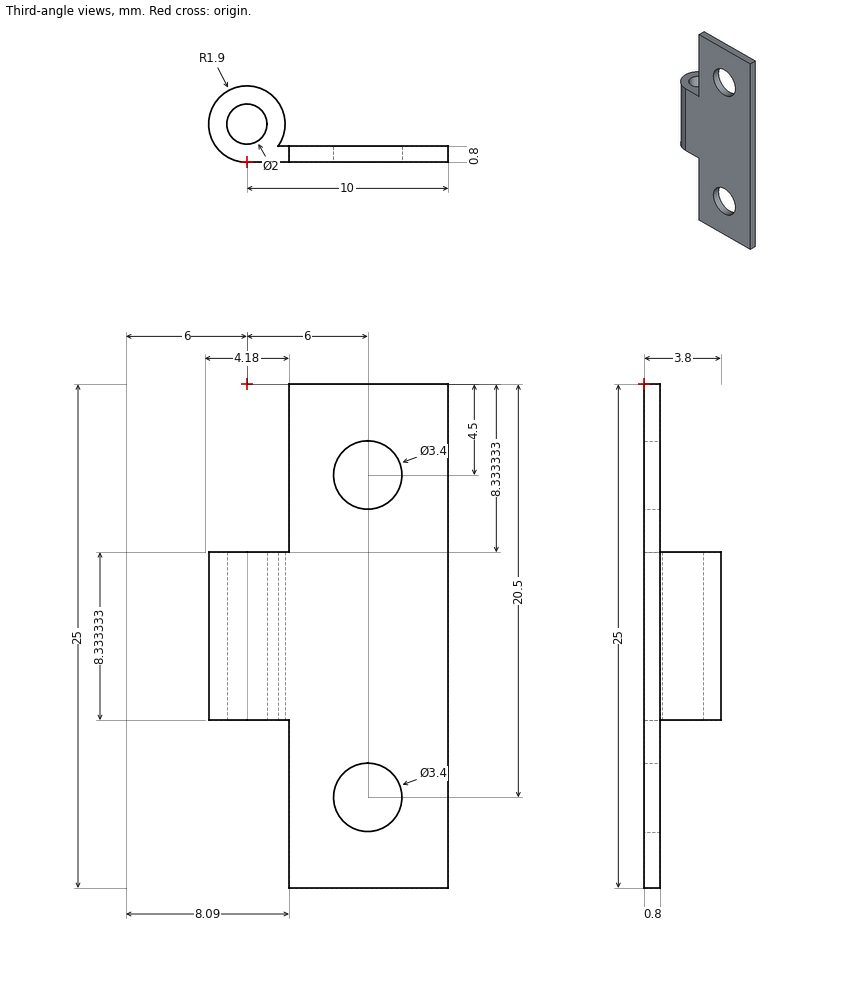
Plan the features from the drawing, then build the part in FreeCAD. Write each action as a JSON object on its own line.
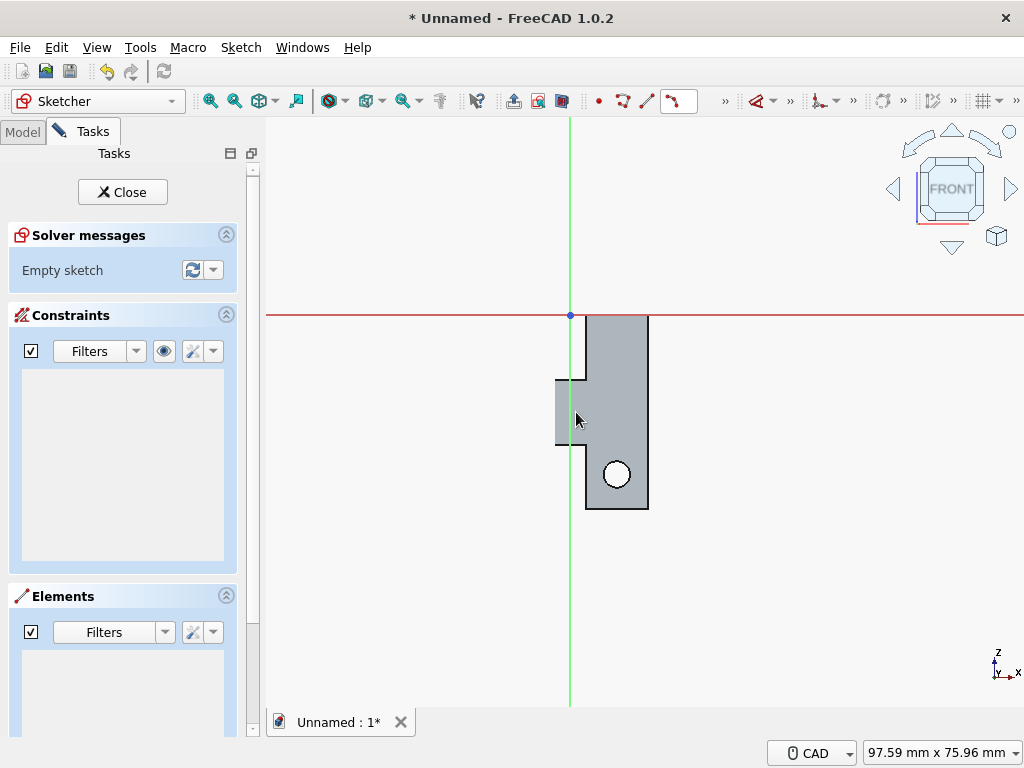
{"action": "scroll", "coordinate": [605, 325], "scroll_direction": "up", "scroll_amount": 9}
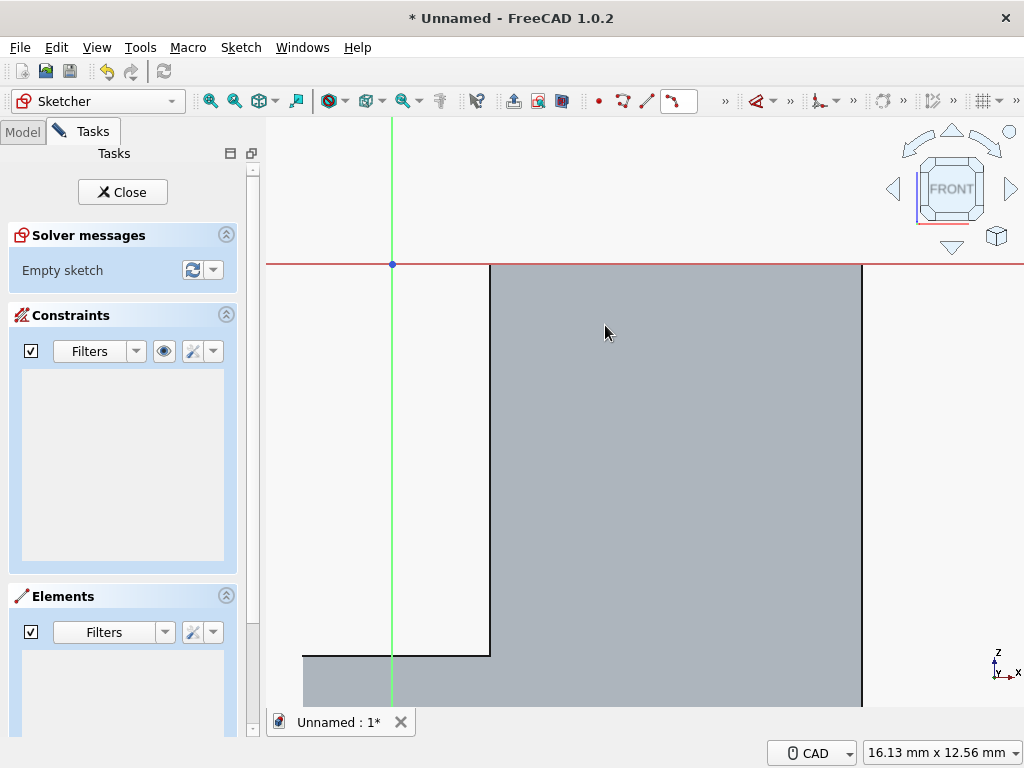
{"action": "key", "text": "g c"}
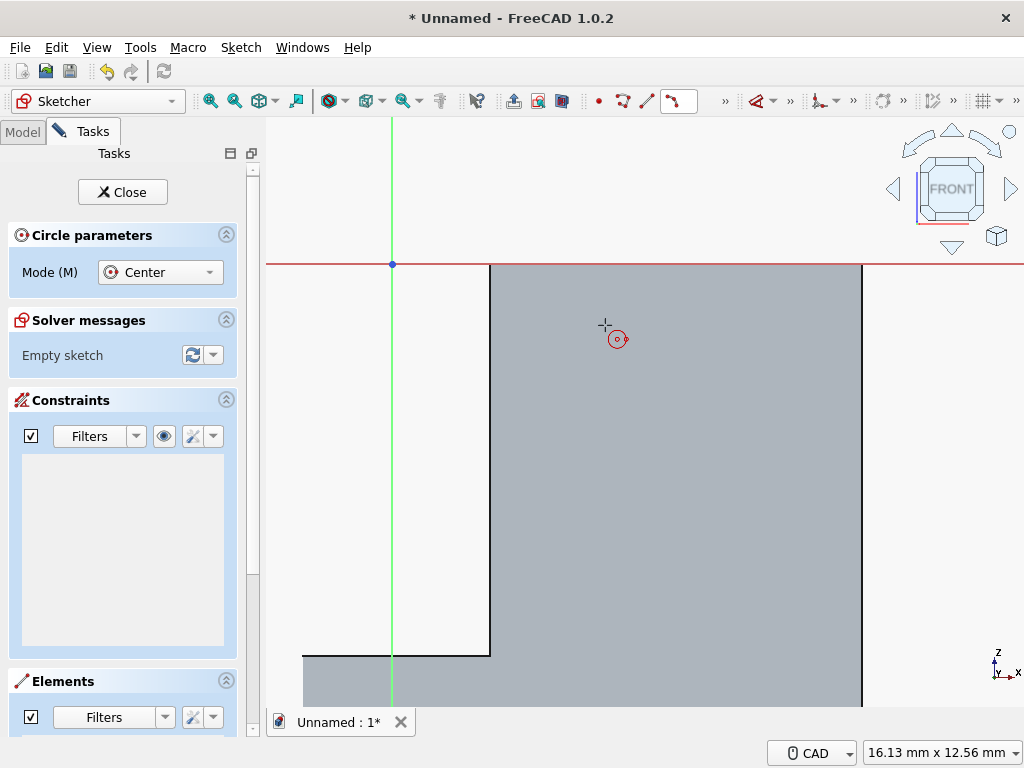
{"action": "left_click", "coordinate": [674, 476]}
{"action": "left_click", "coordinate": [730, 419]}
{"action": "key", "text": "Escape"}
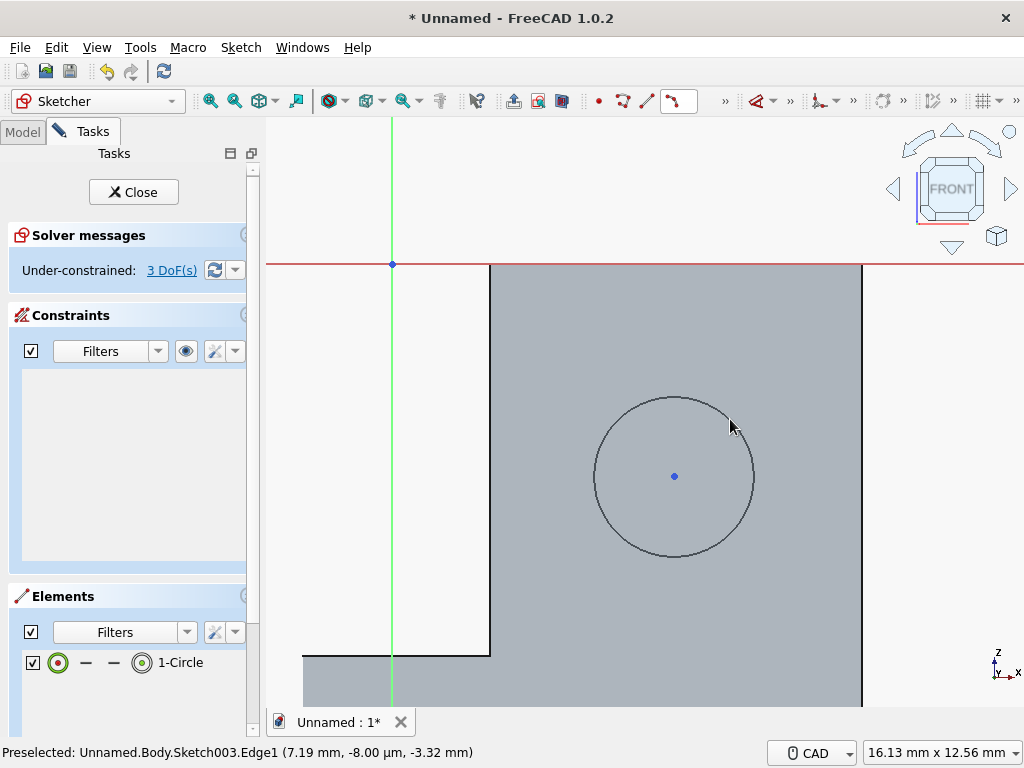
{"action": "left_click", "coordinate": [756, 102]}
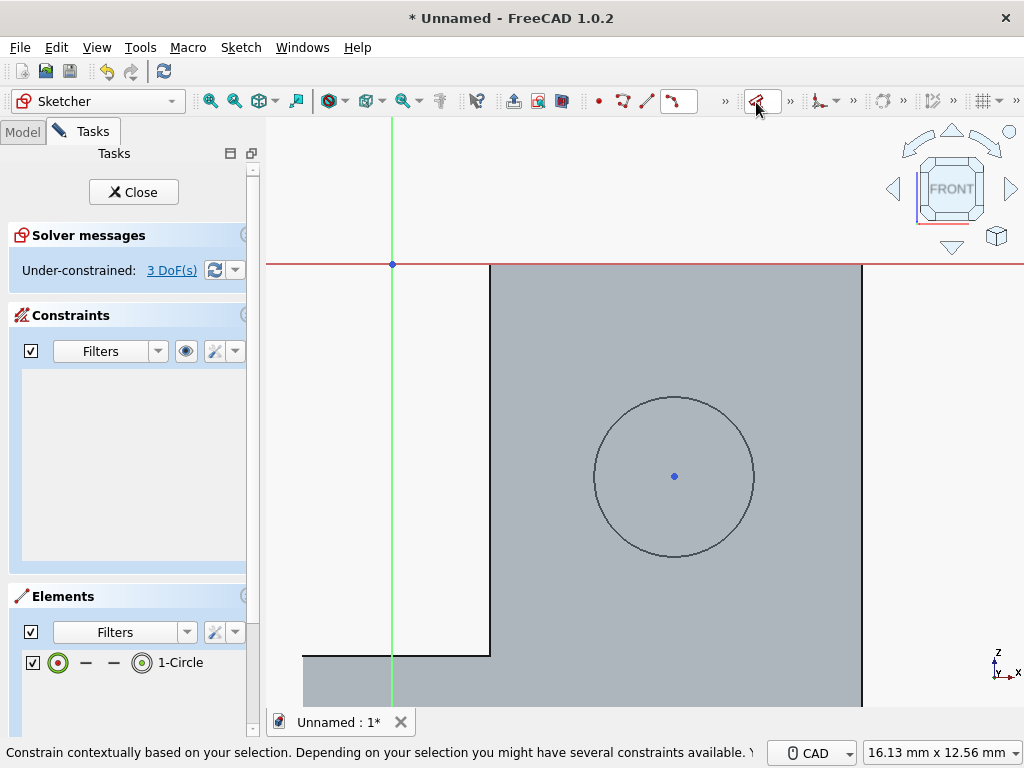
{"action": "left_click", "coordinate": [730, 420]}
{"action": "left_click", "coordinate": [752, 397]}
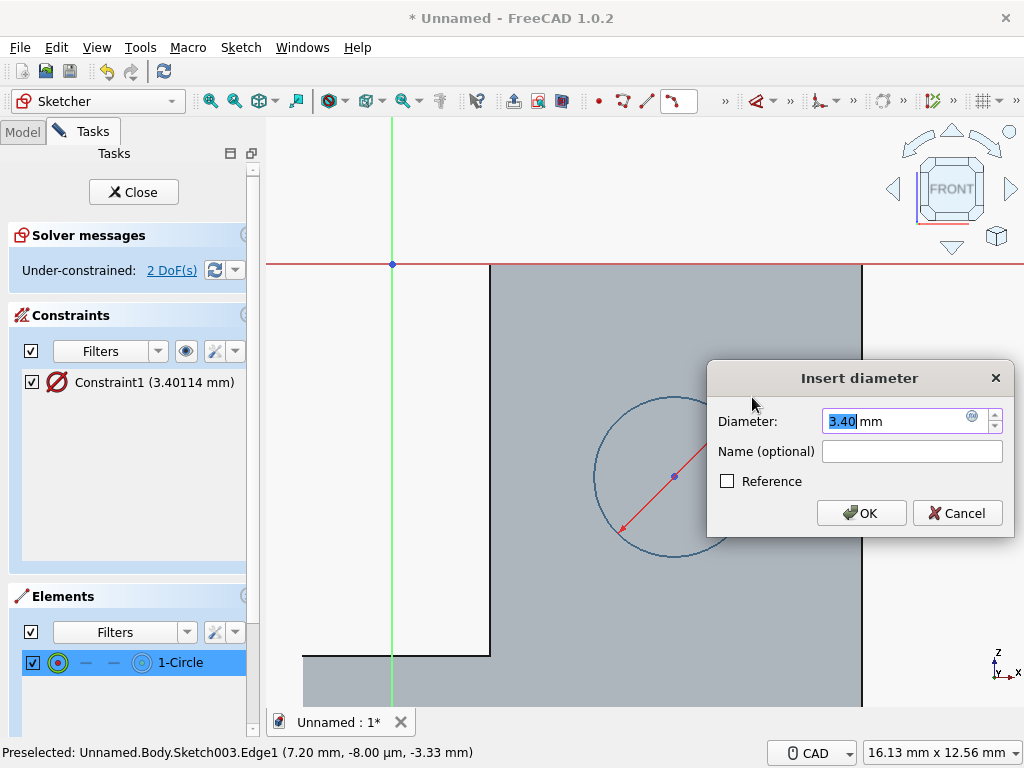
{"action": "type", "text": "3.4"}
{"action": "key", "text": "Return"}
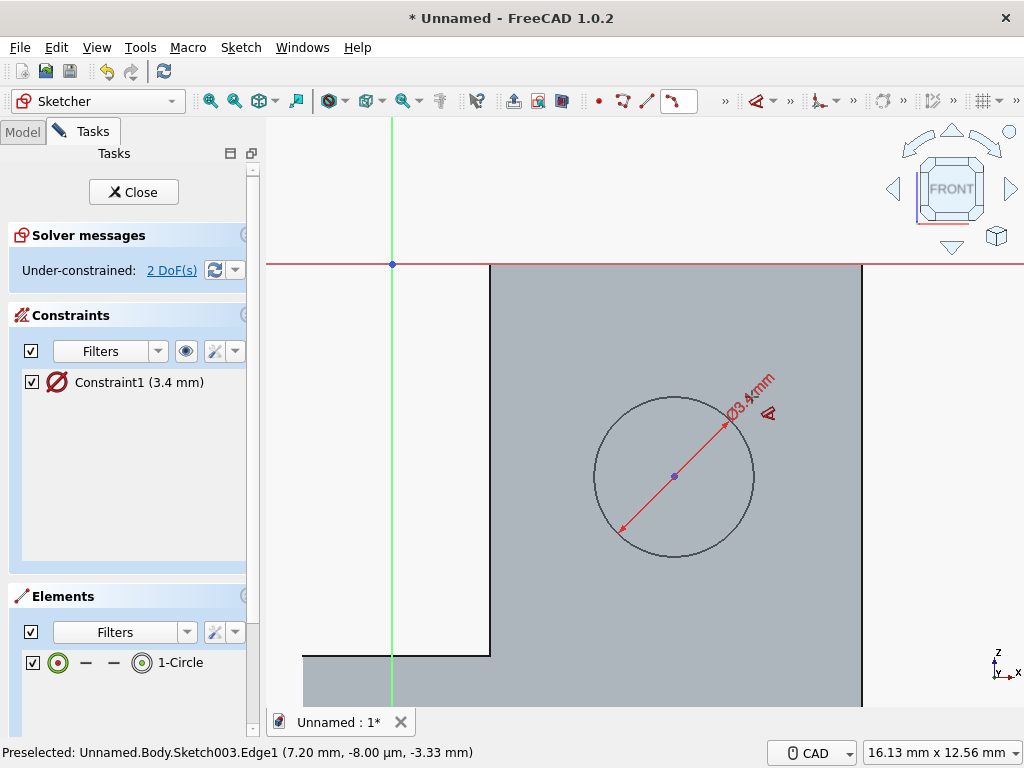
{"action": "left_click", "coordinate": [674, 477]}
{"action": "left_click", "coordinate": [533, 230]}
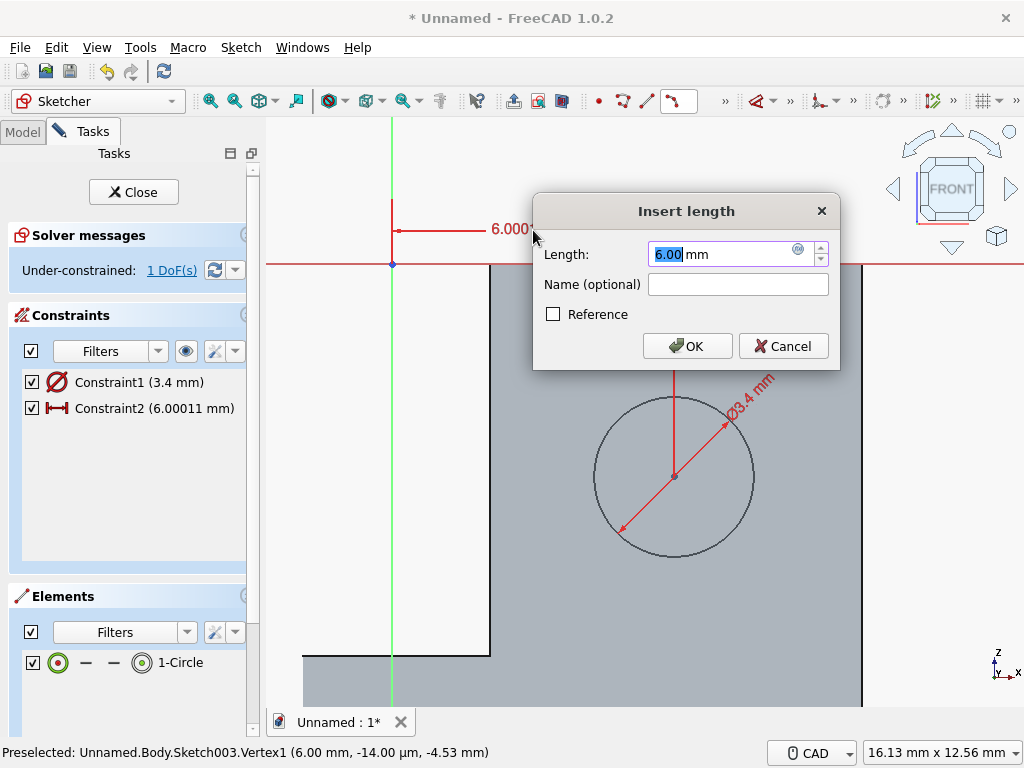
{"action": "type", "text": "6"}
{"action": "key", "text": "Return"}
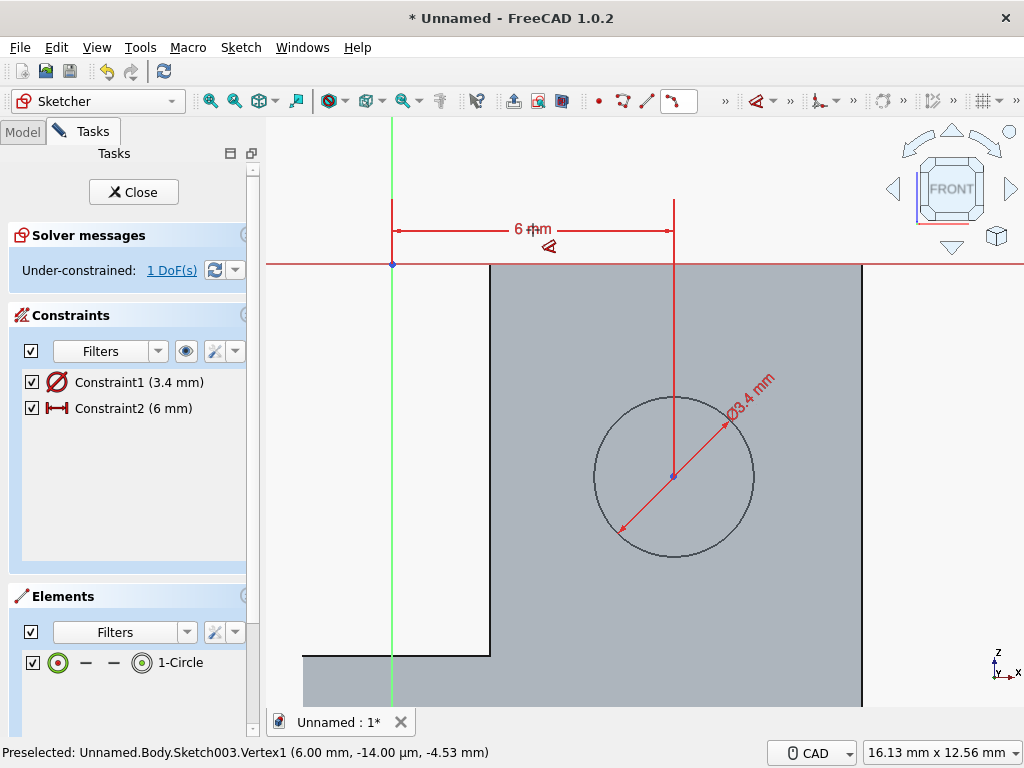
{"action": "left_click", "coordinate": [674, 477]}
{"action": "left_click", "coordinate": [358, 371]}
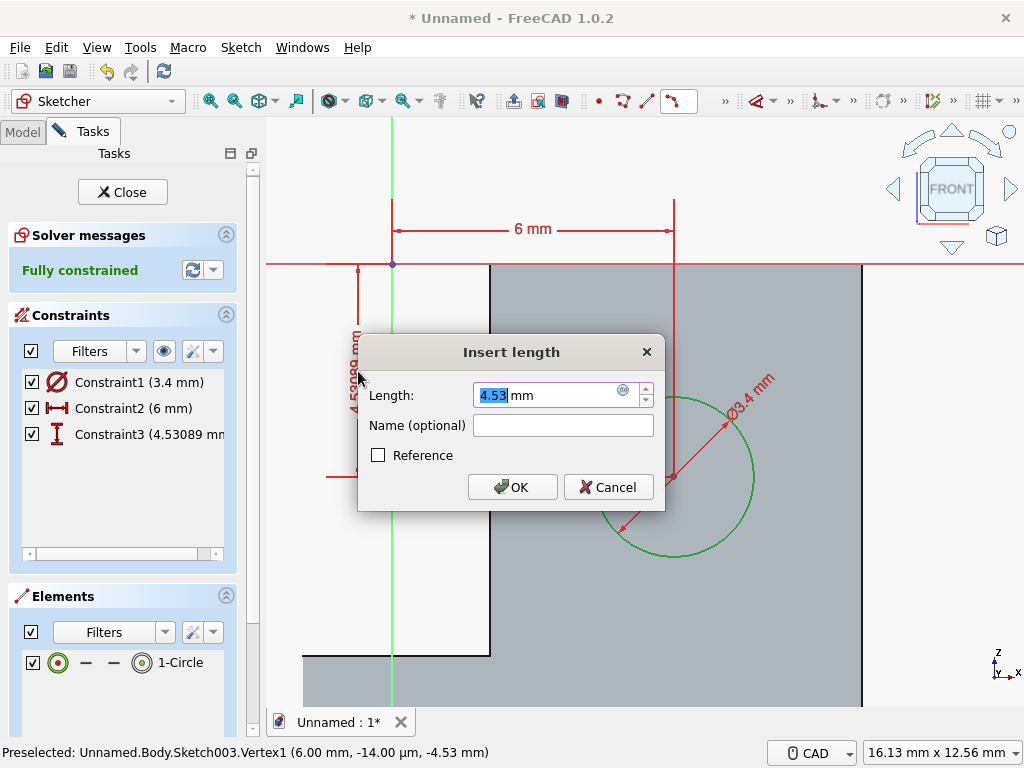
{"action": "type", "text": "4.5"}
{"action": "key", "text": "Return"}
{"action": "key", "text": "Escape"}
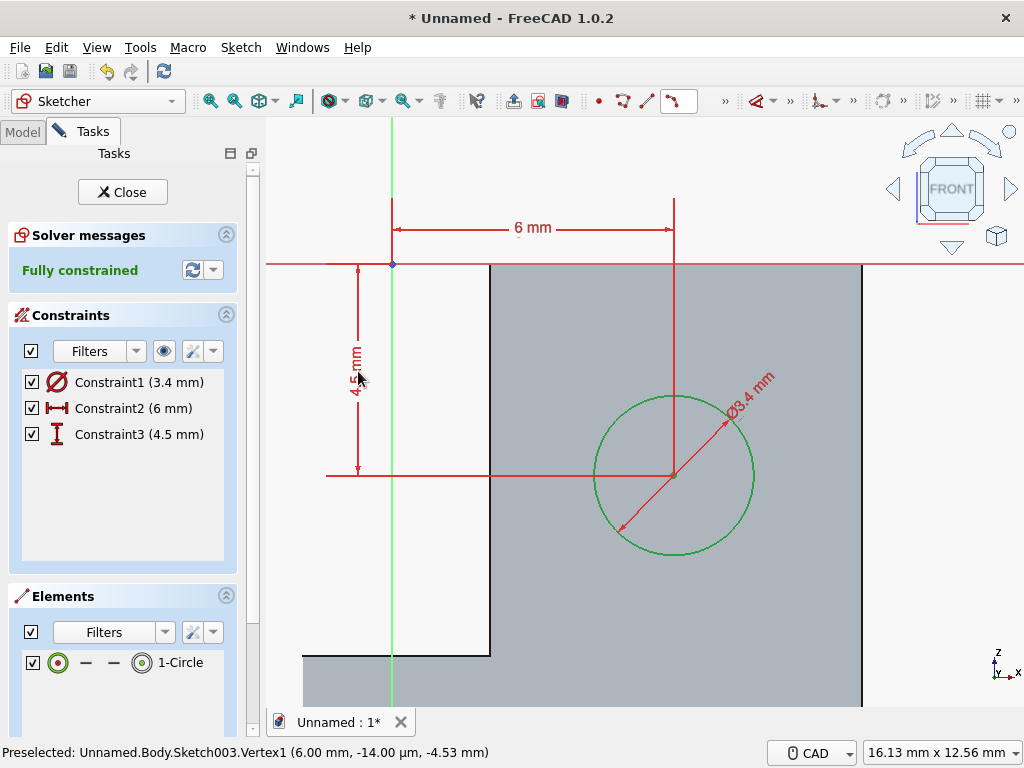
{"action": "left_click", "coordinate": [123, 192]}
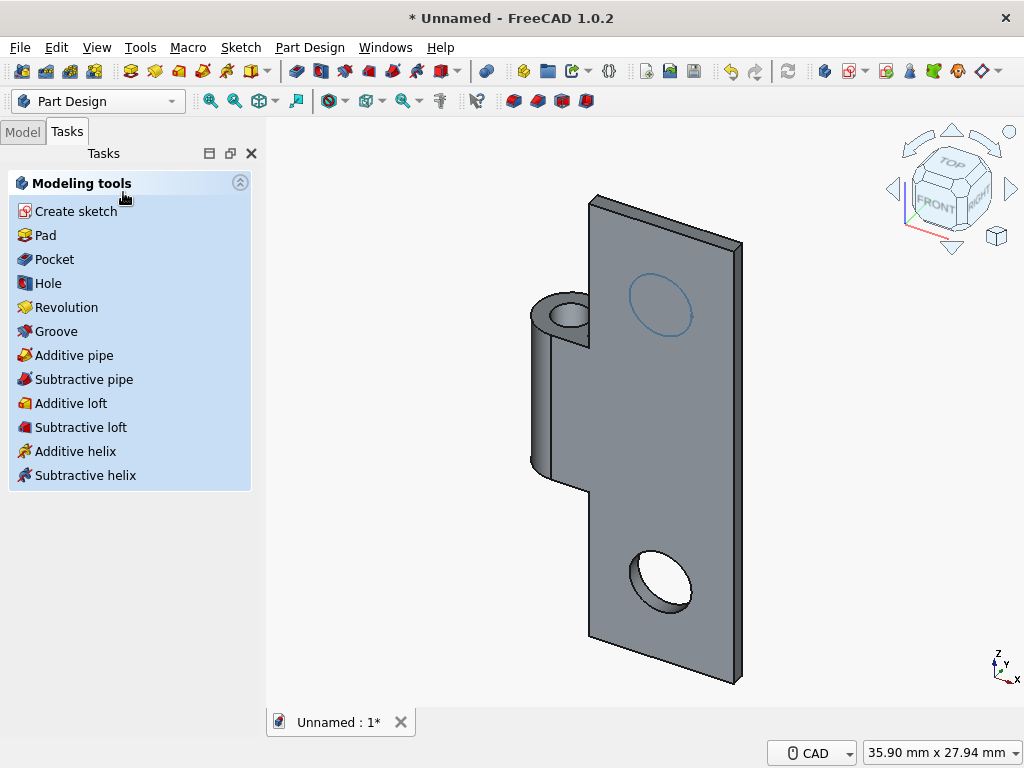
{"action": "left_click", "coordinate": [298, 72]}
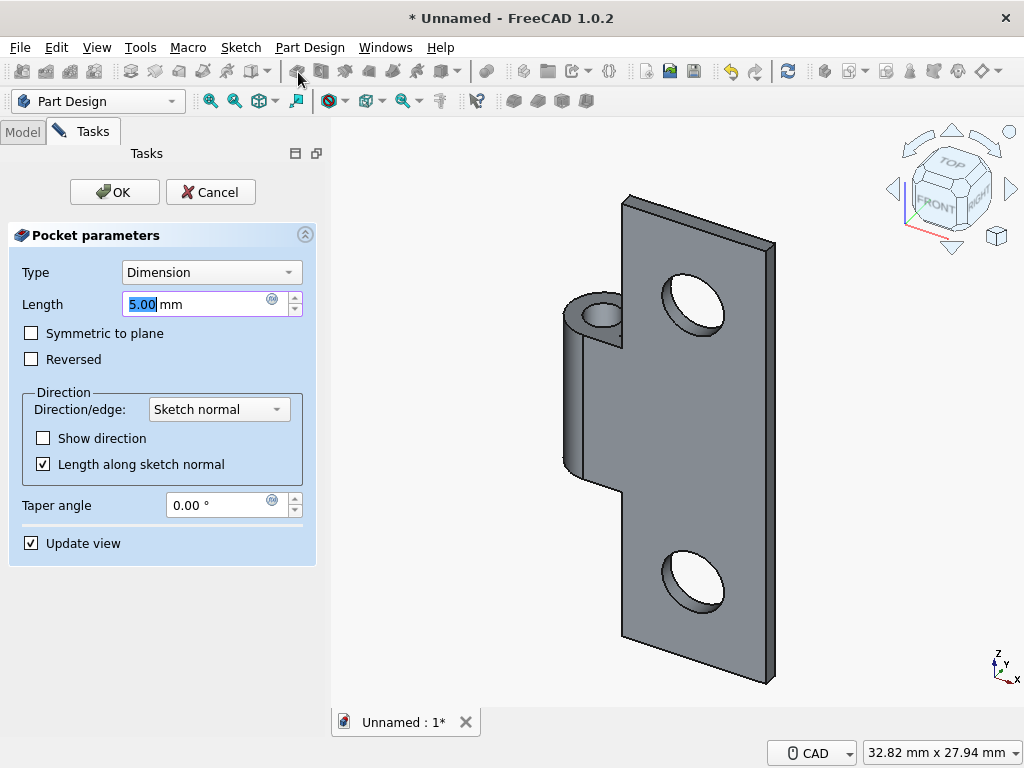
{"action": "type", "text": "0.8"}
{"action": "key", "text": "Tab"}